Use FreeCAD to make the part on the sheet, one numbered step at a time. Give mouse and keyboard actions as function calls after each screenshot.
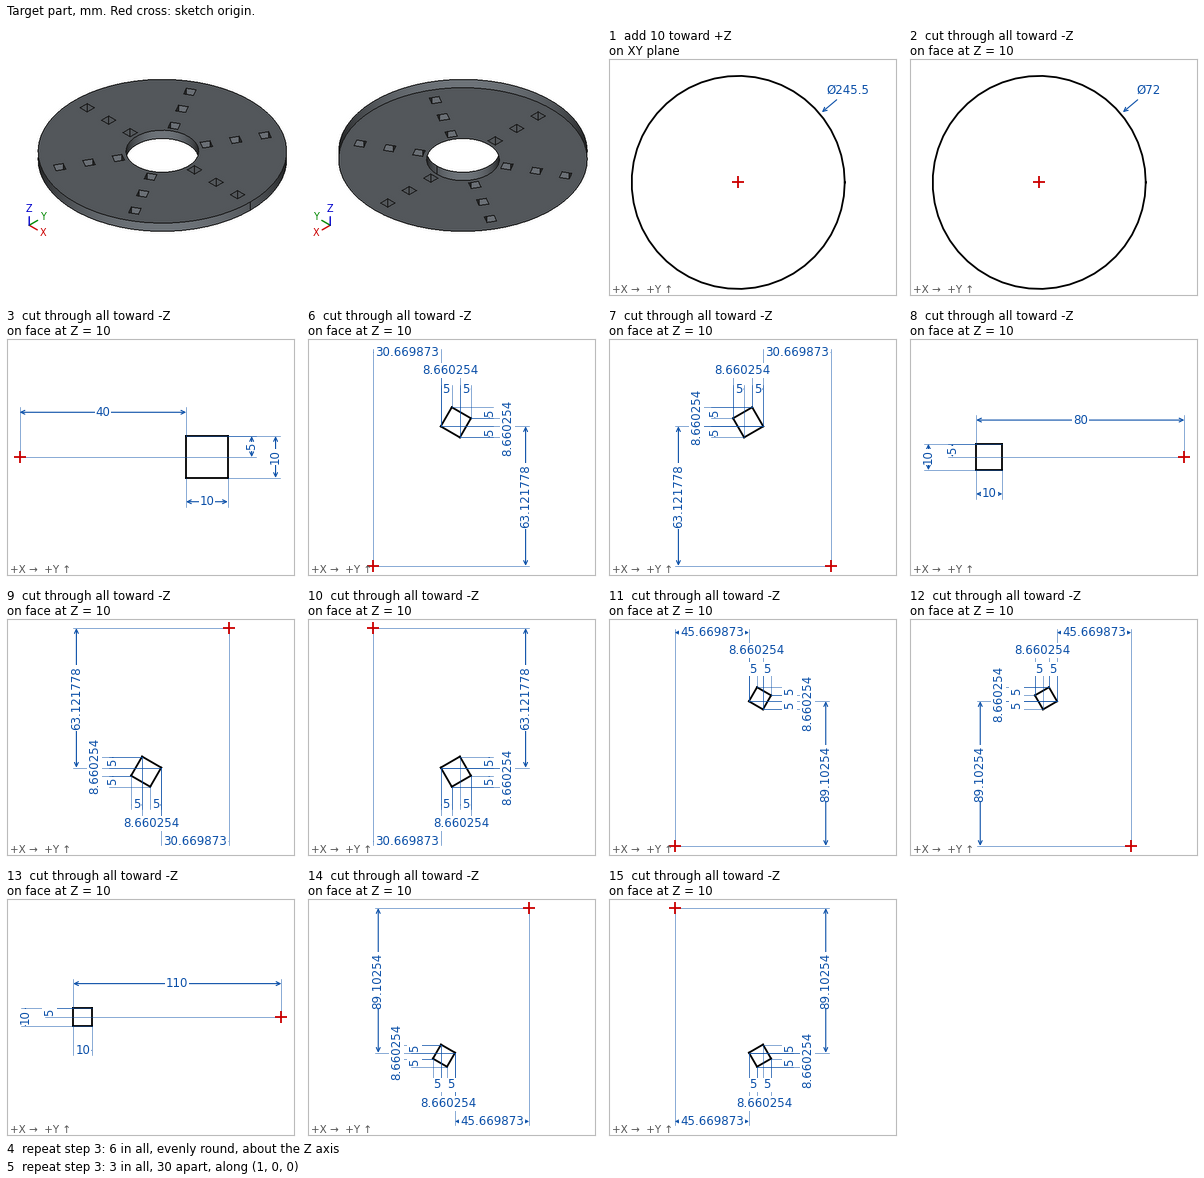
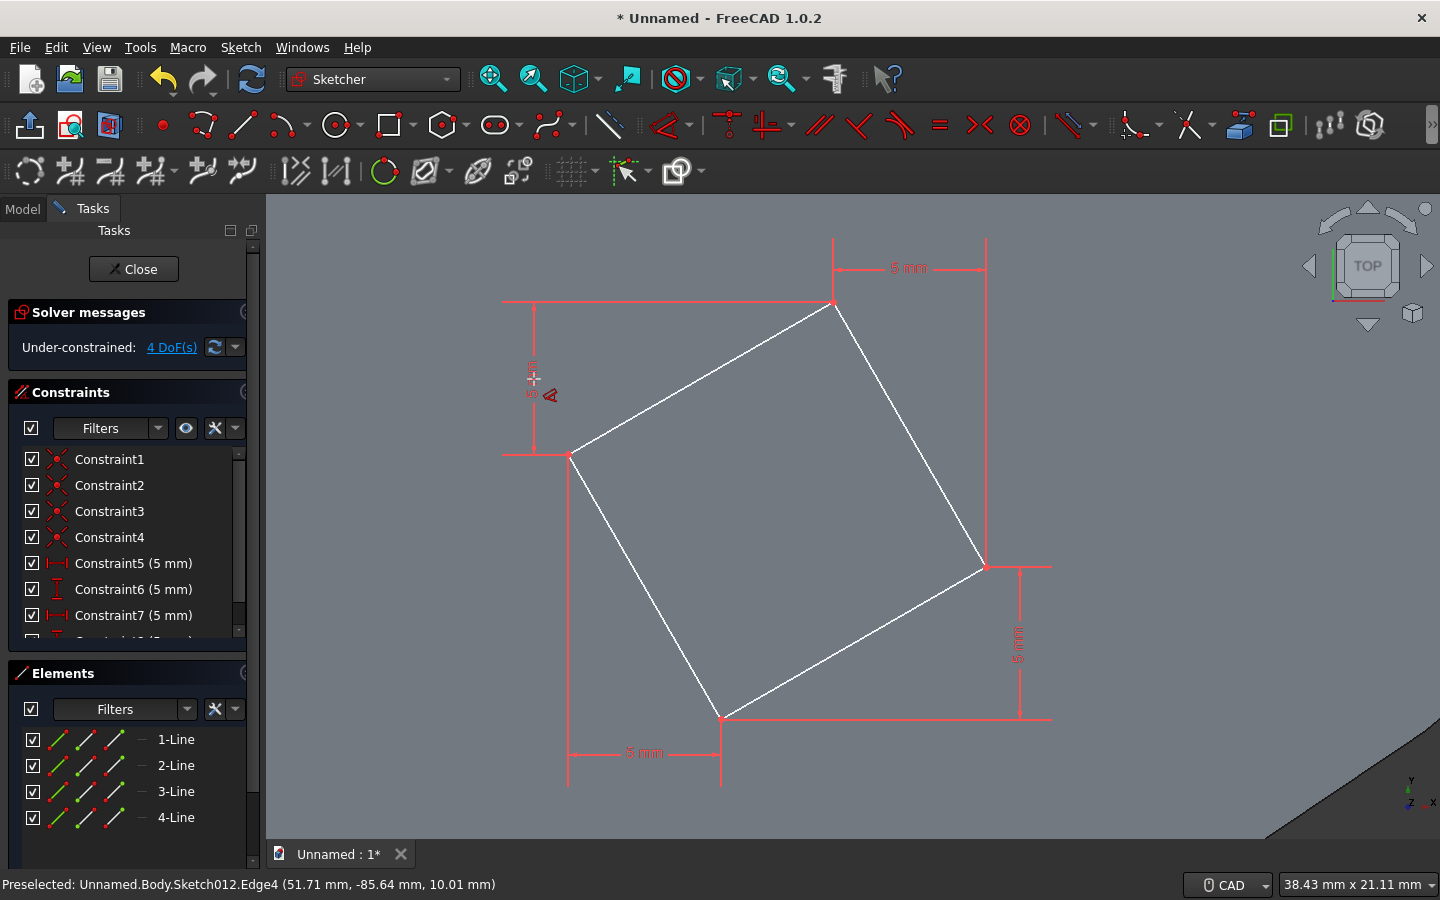
click(568, 455)
click(602, 338)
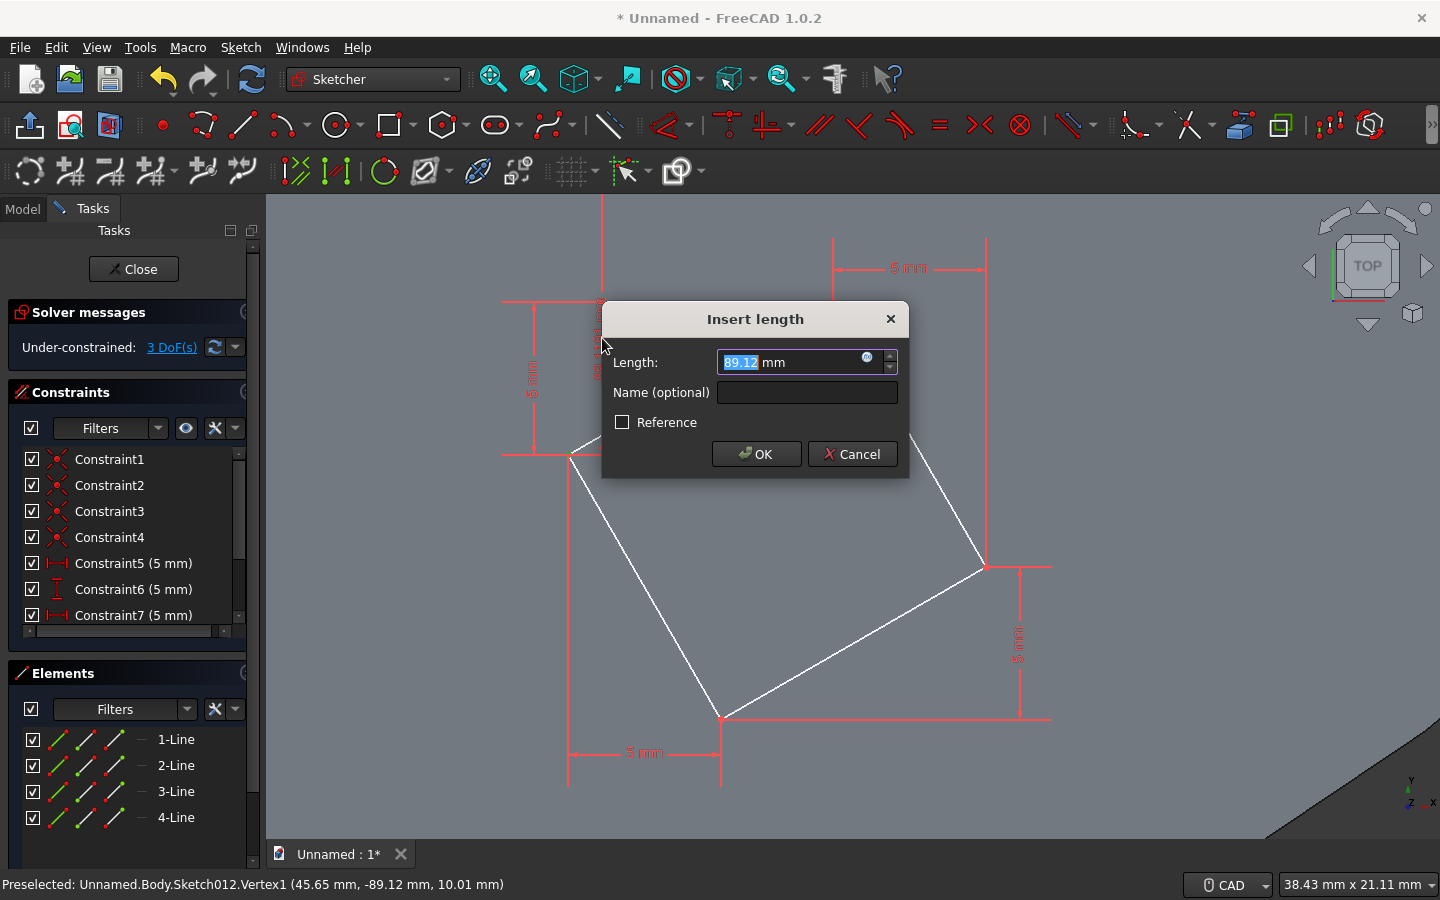
text(89.10254)
key(Return)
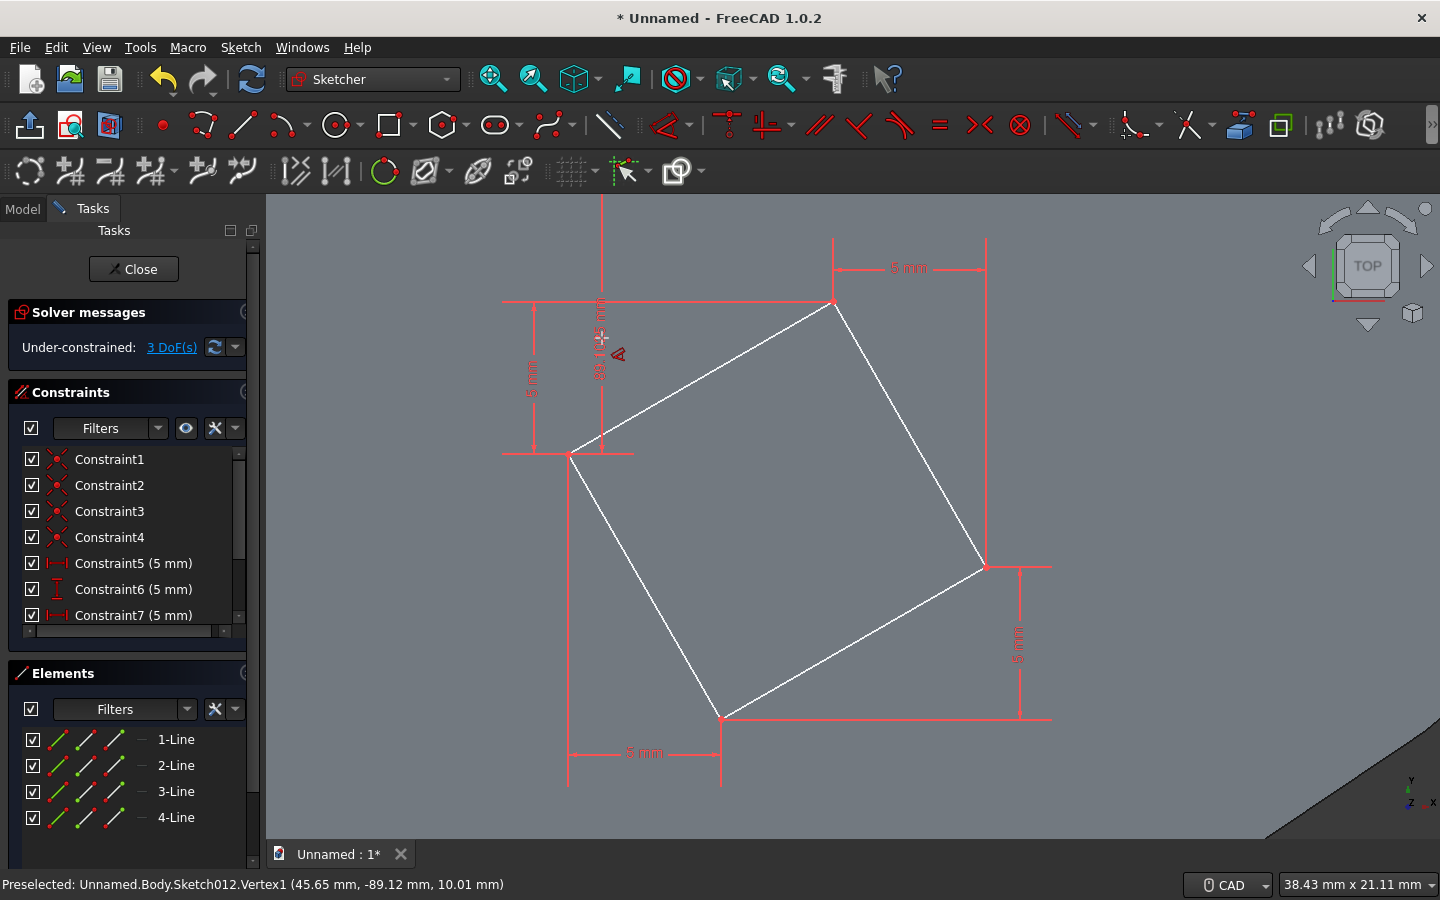
click(614, 534)
click(534, 587)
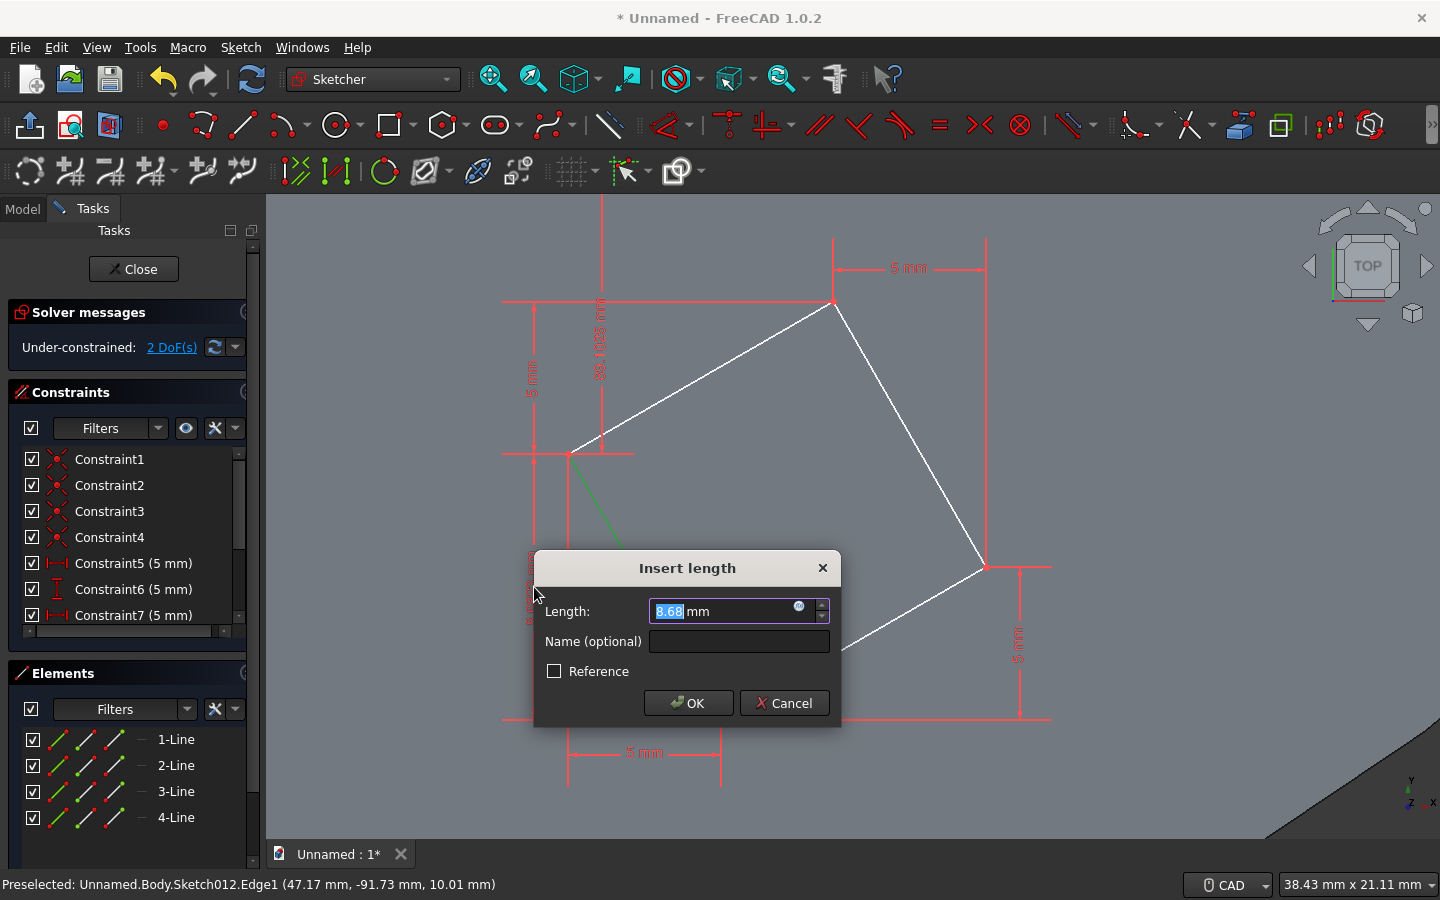
text(8.660254)
key(Return)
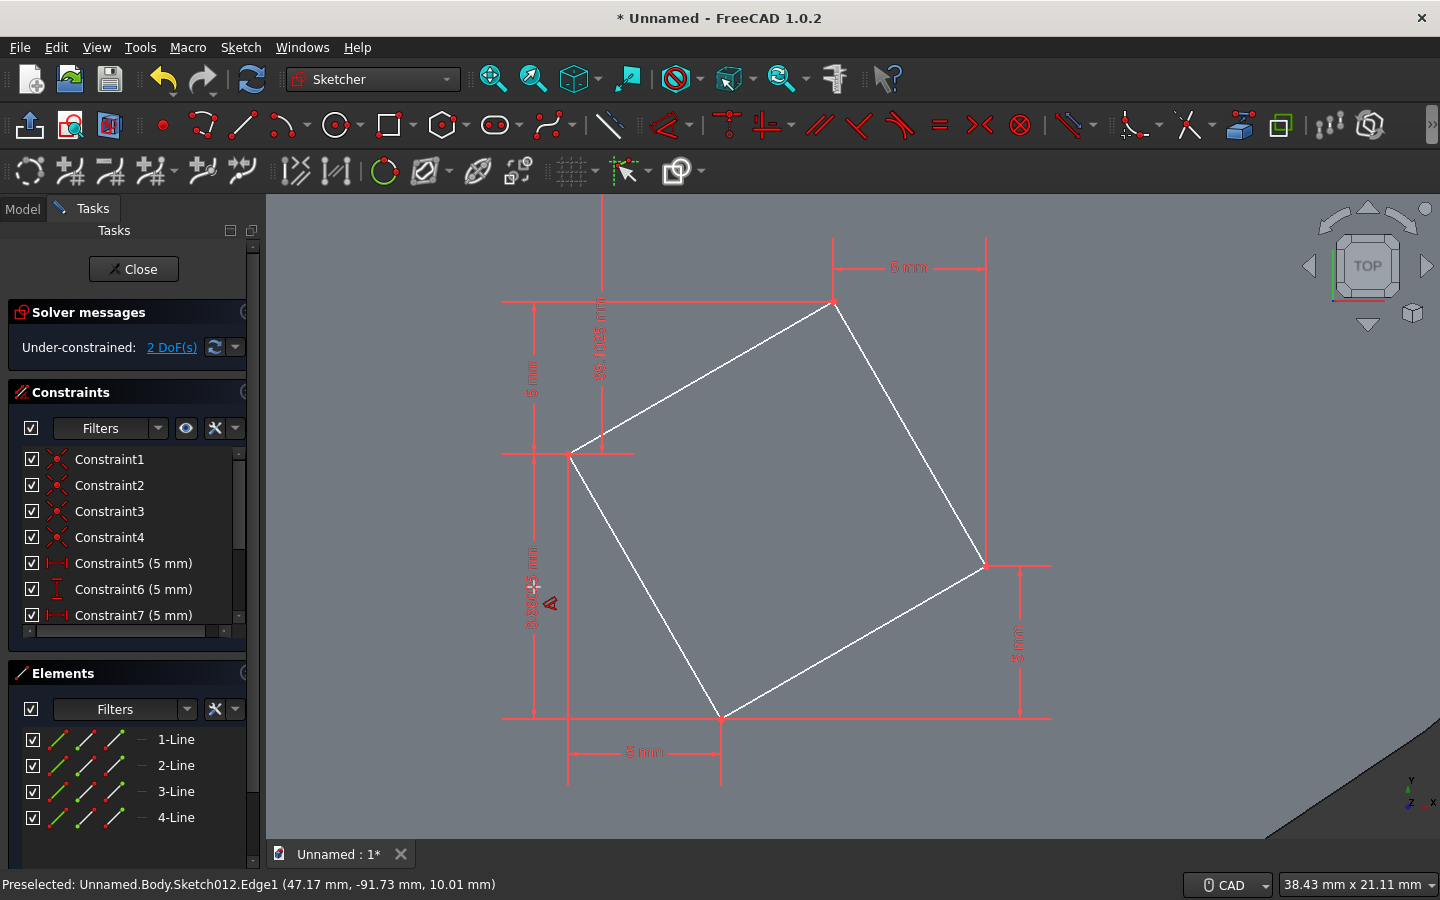
click(801, 673)
click(854, 753)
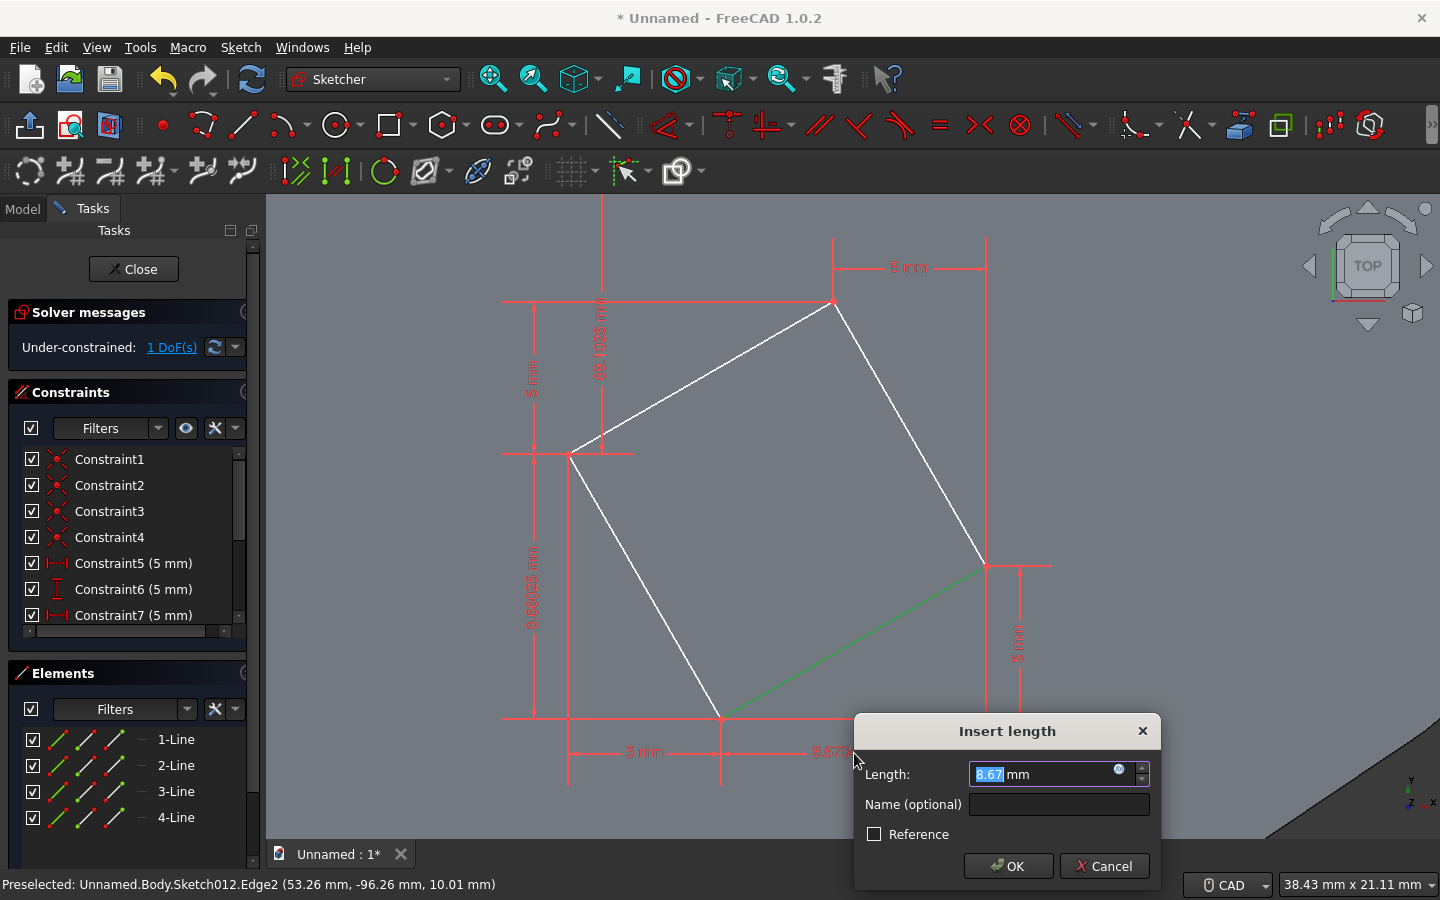
text(8.660254)
key(Return)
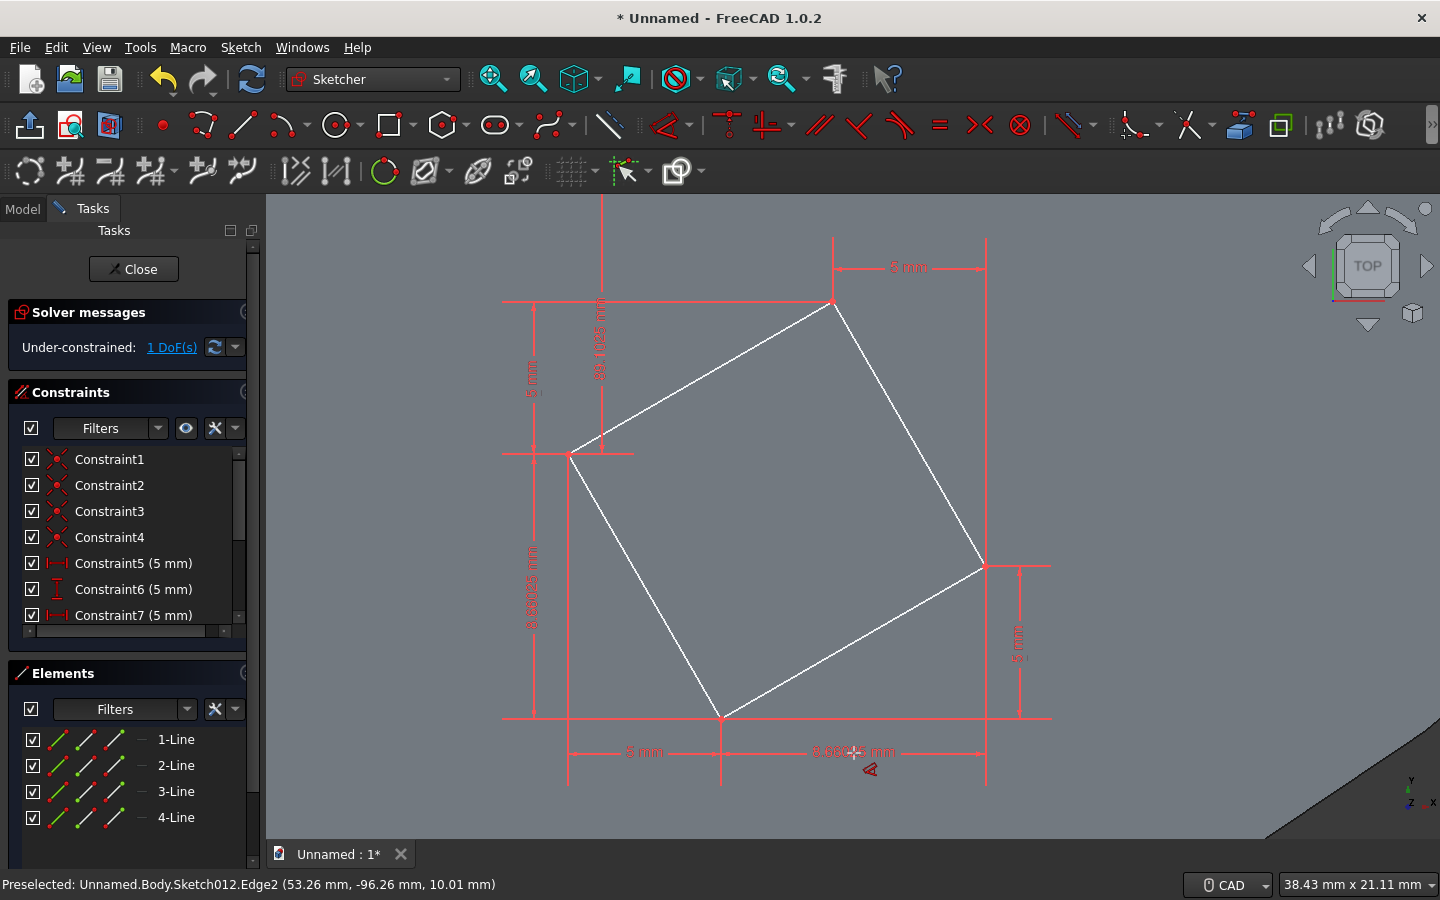
click(568, 454)
click(431, 488)